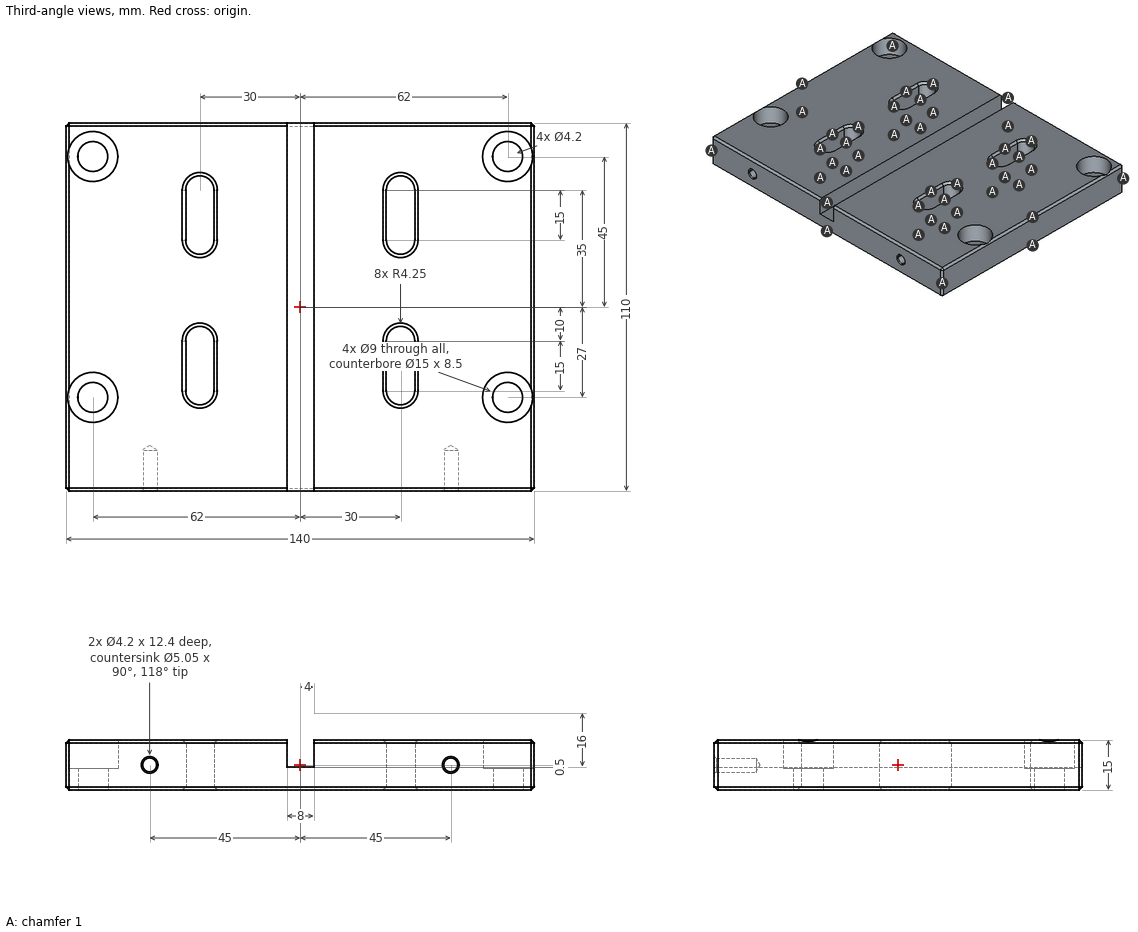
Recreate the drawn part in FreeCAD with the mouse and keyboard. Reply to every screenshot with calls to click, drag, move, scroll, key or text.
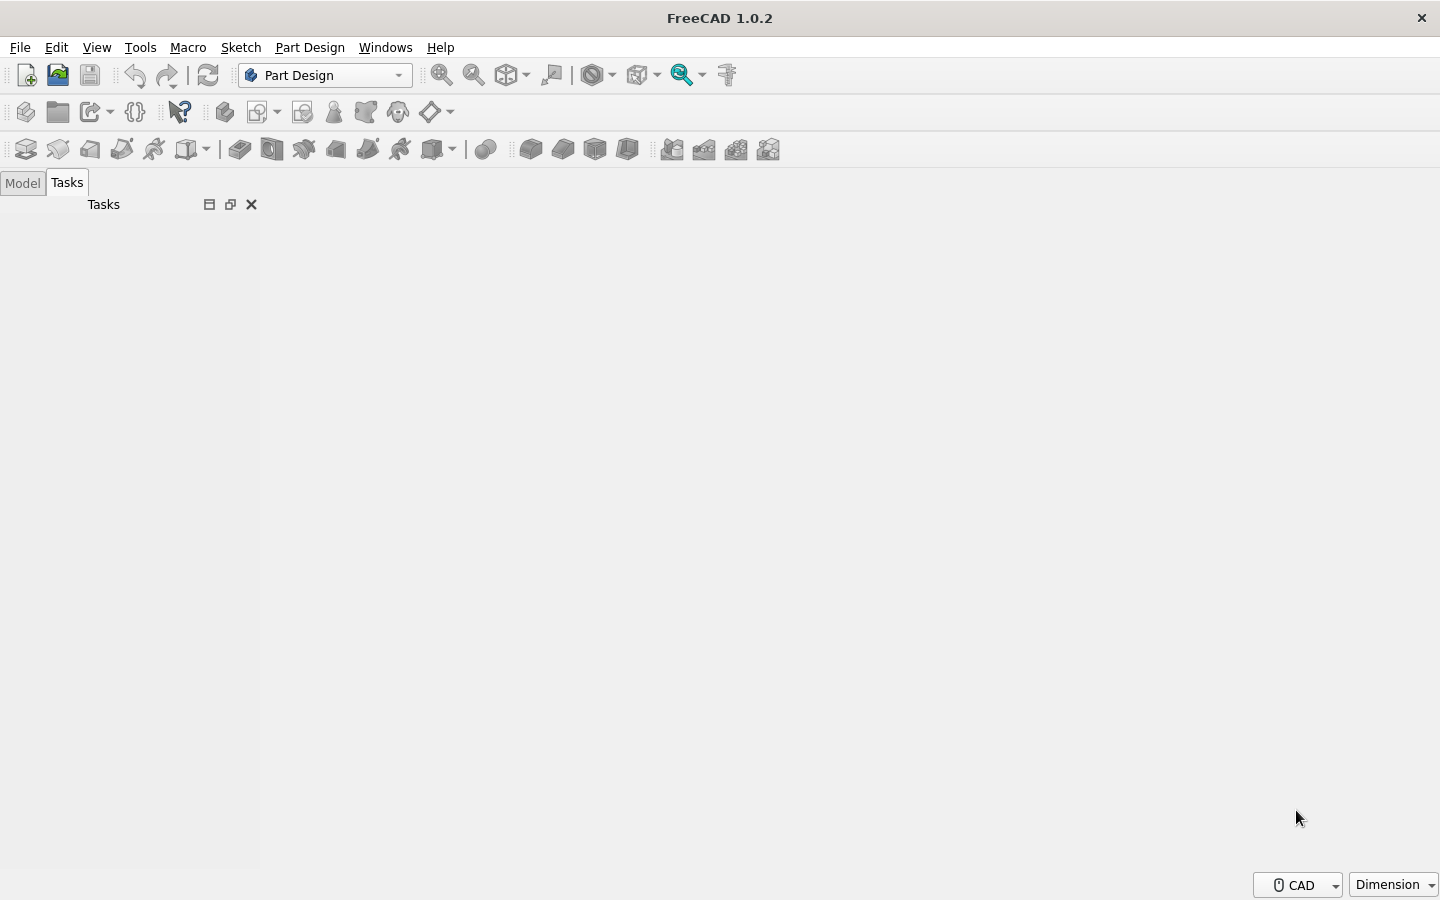
key(ctrl+n)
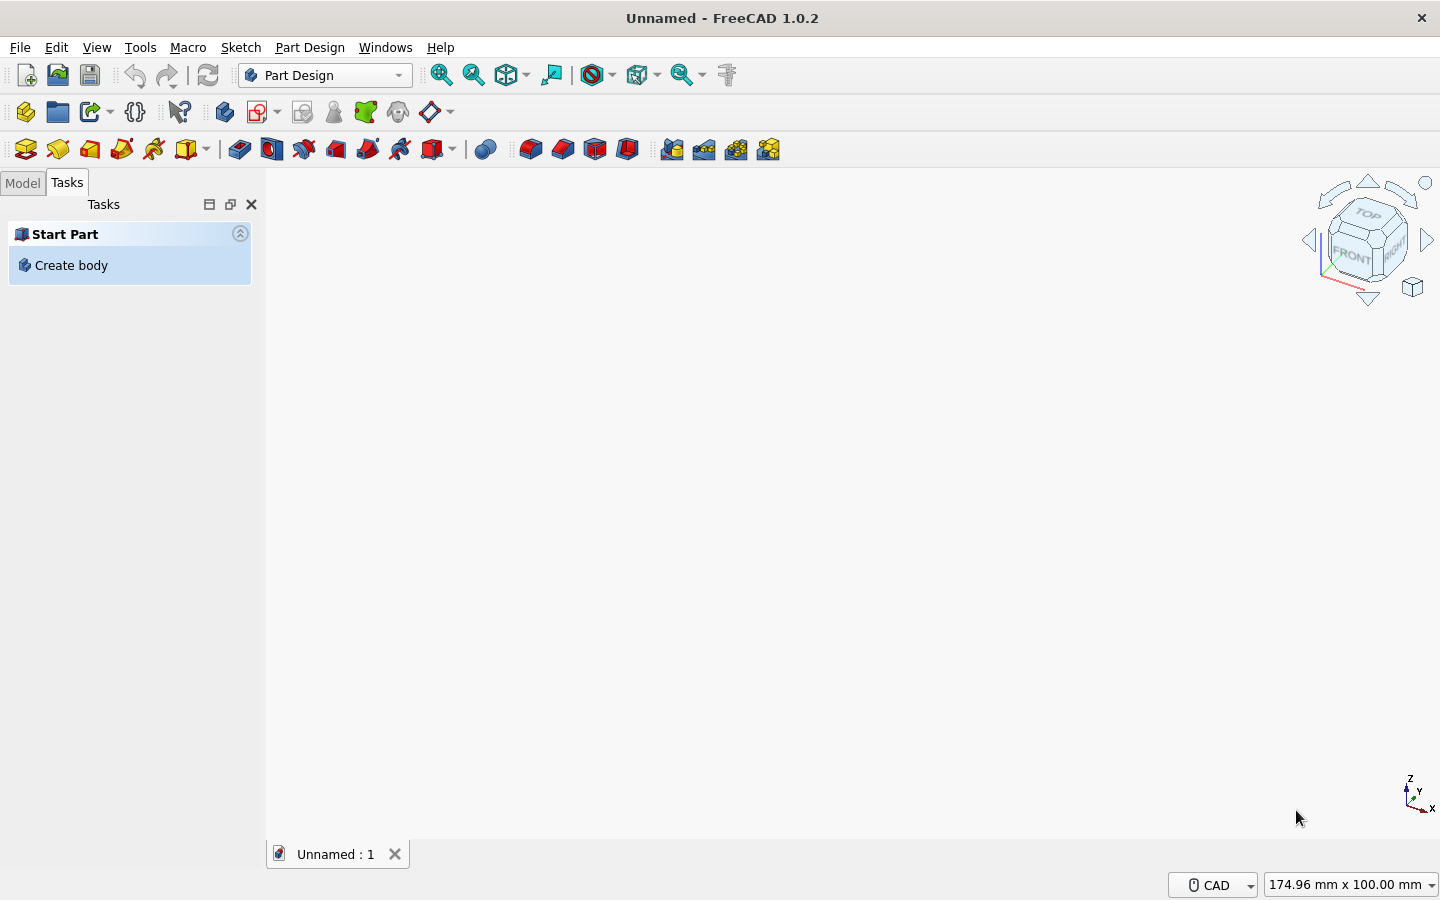
click(258, 112)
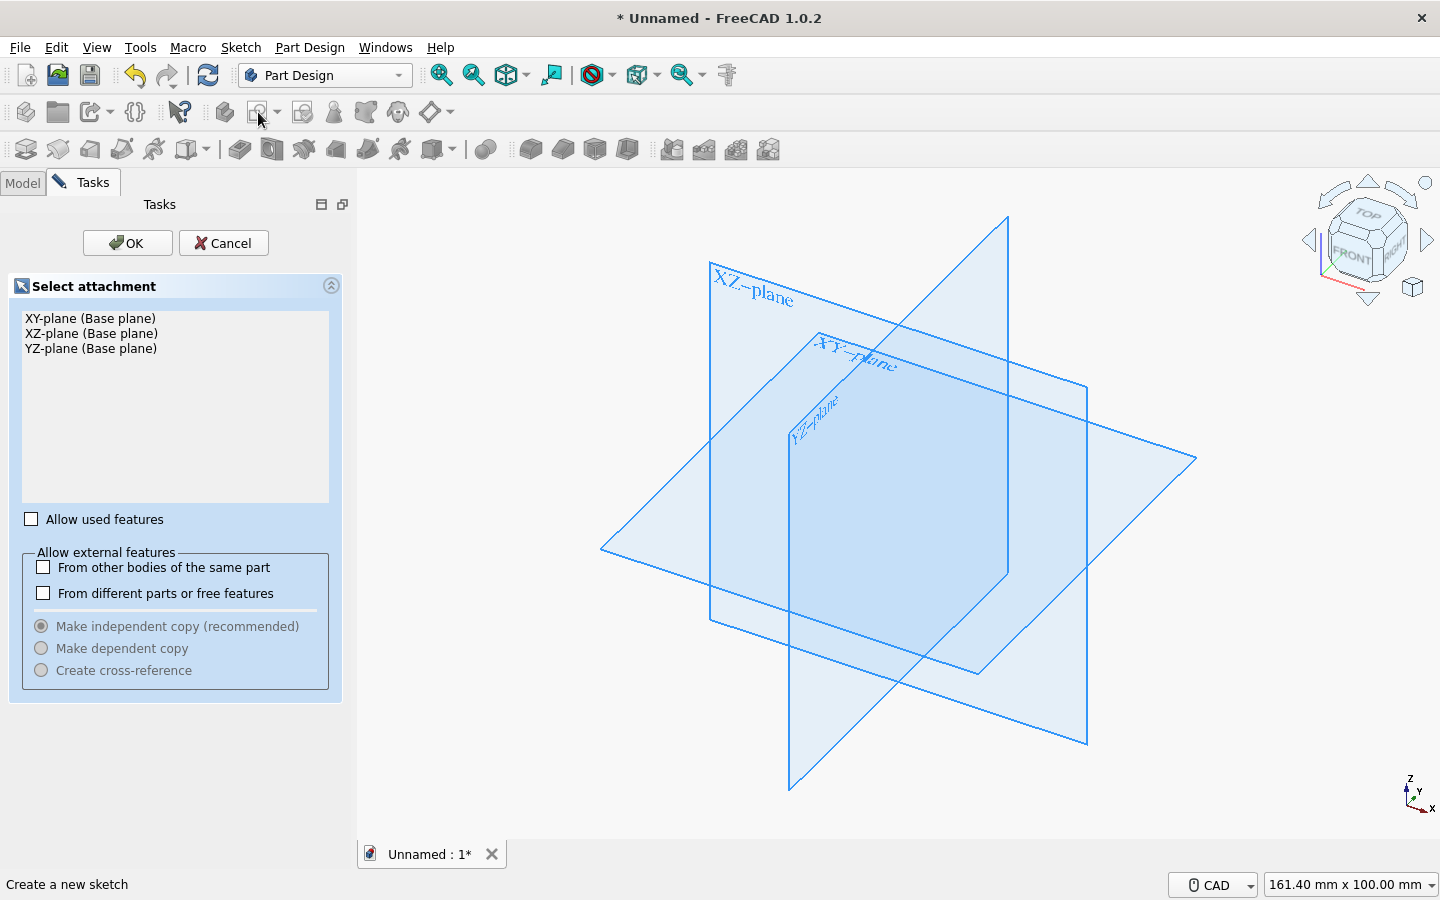
click(82, 318)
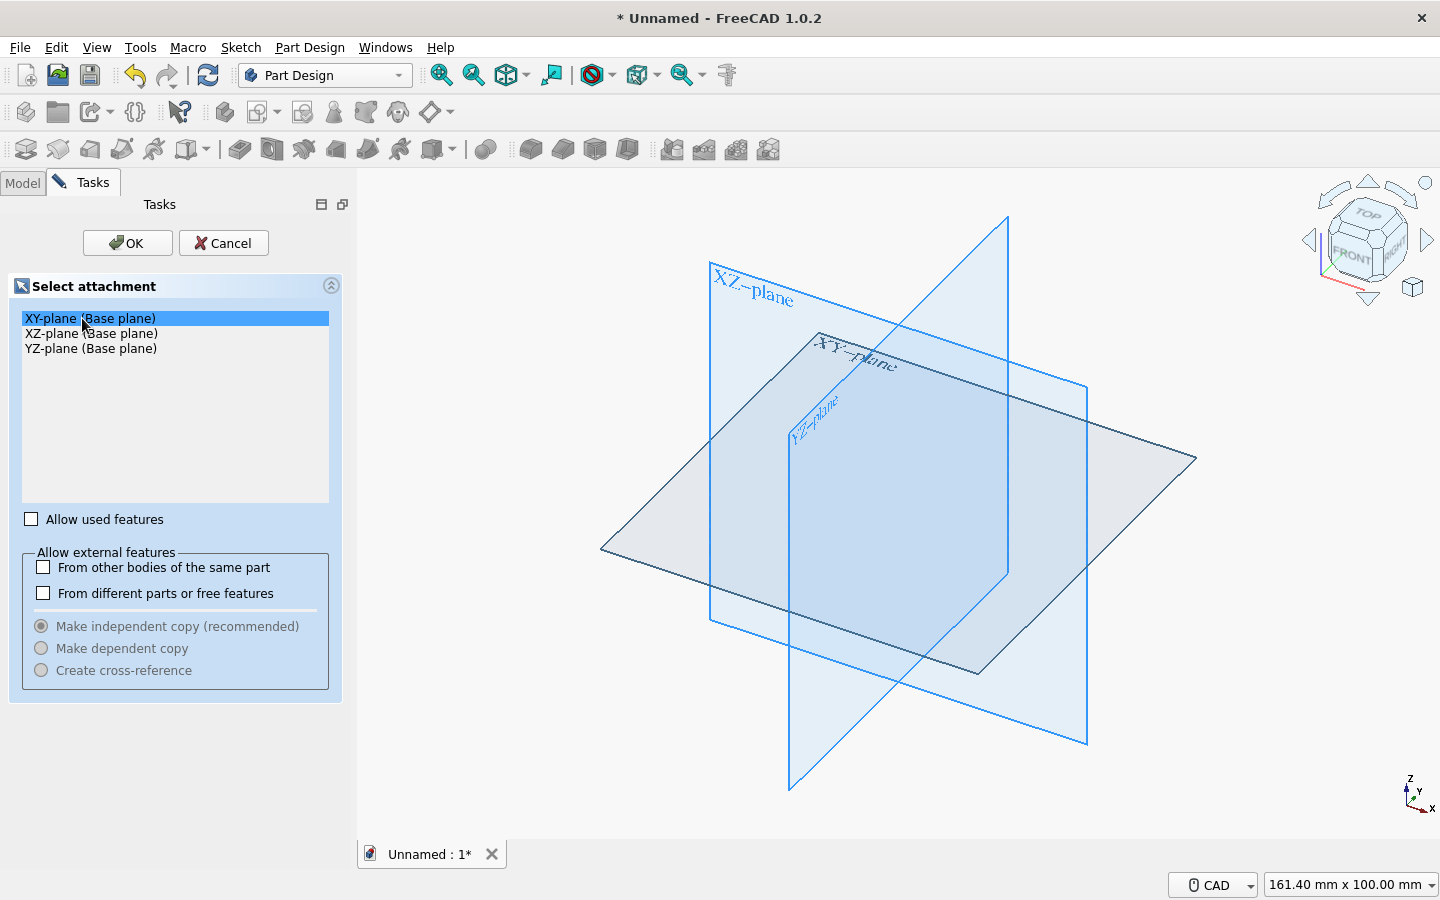
click(128, 243)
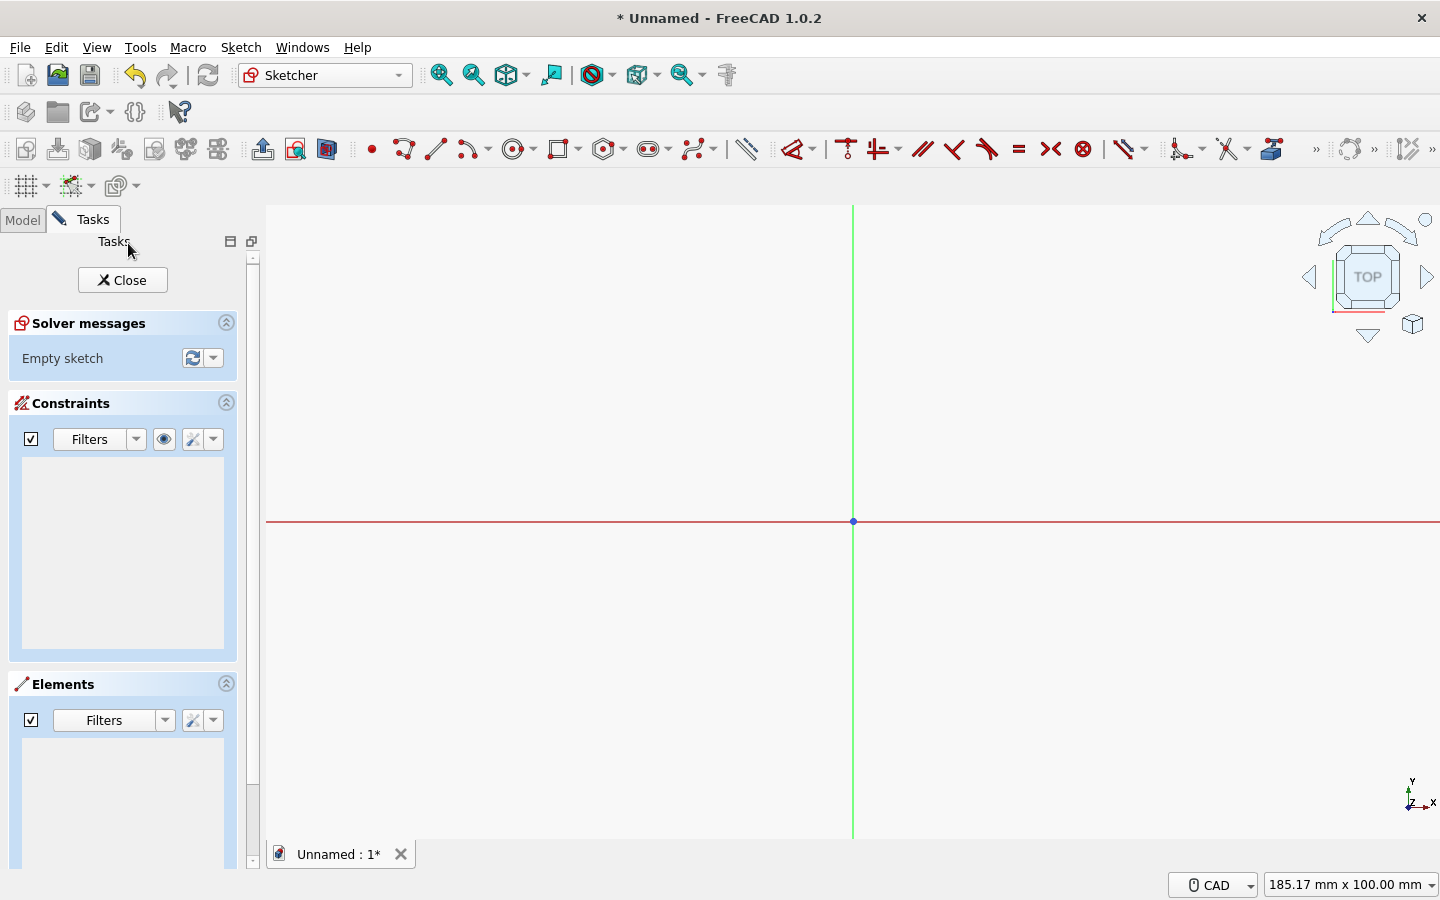
scroll(701, 522, down, 3)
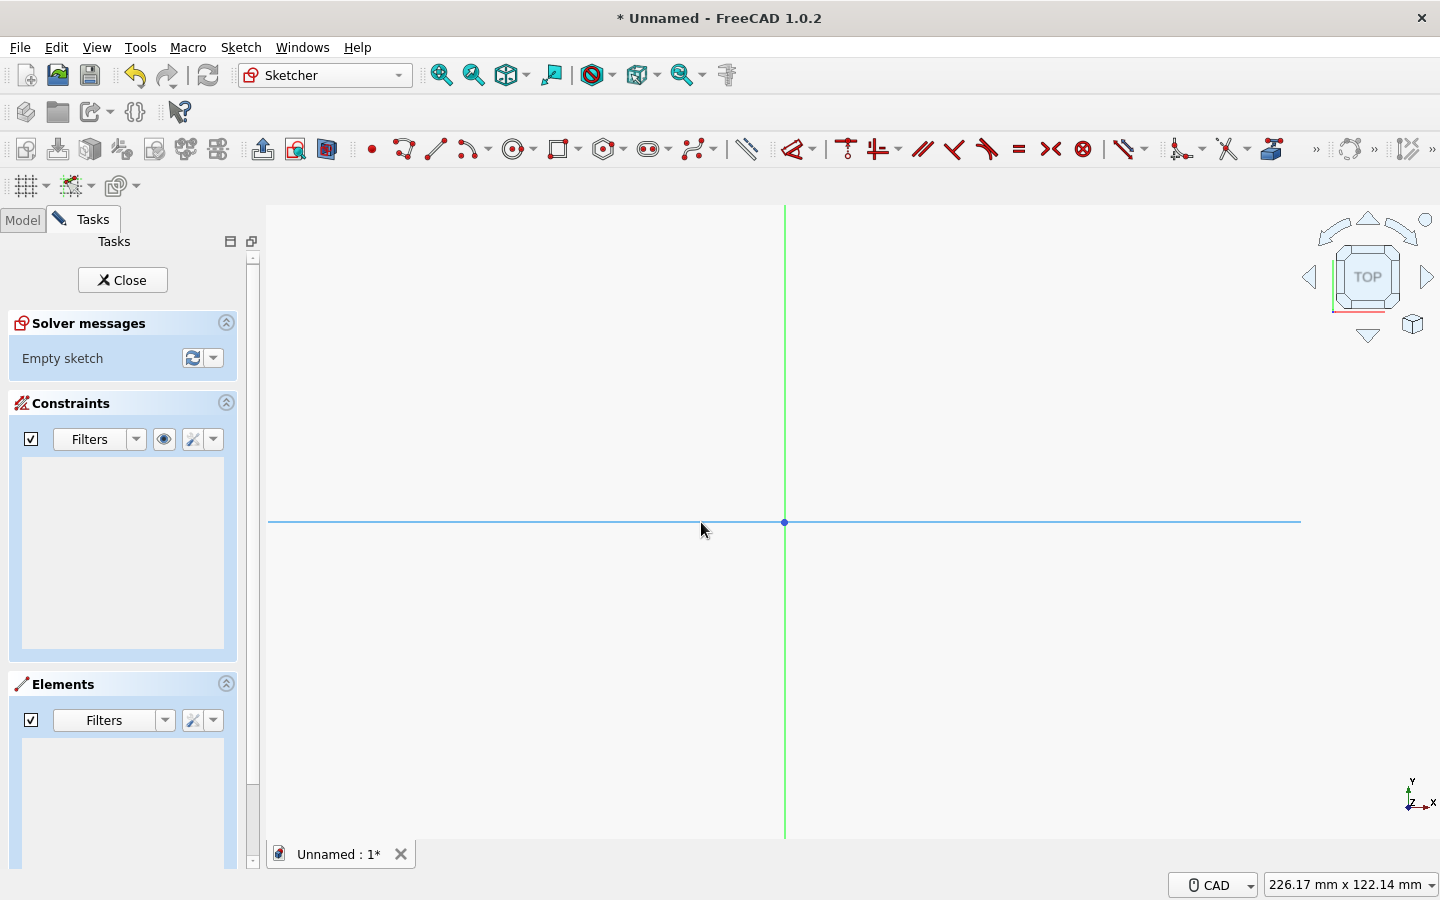
key(g)
key(v)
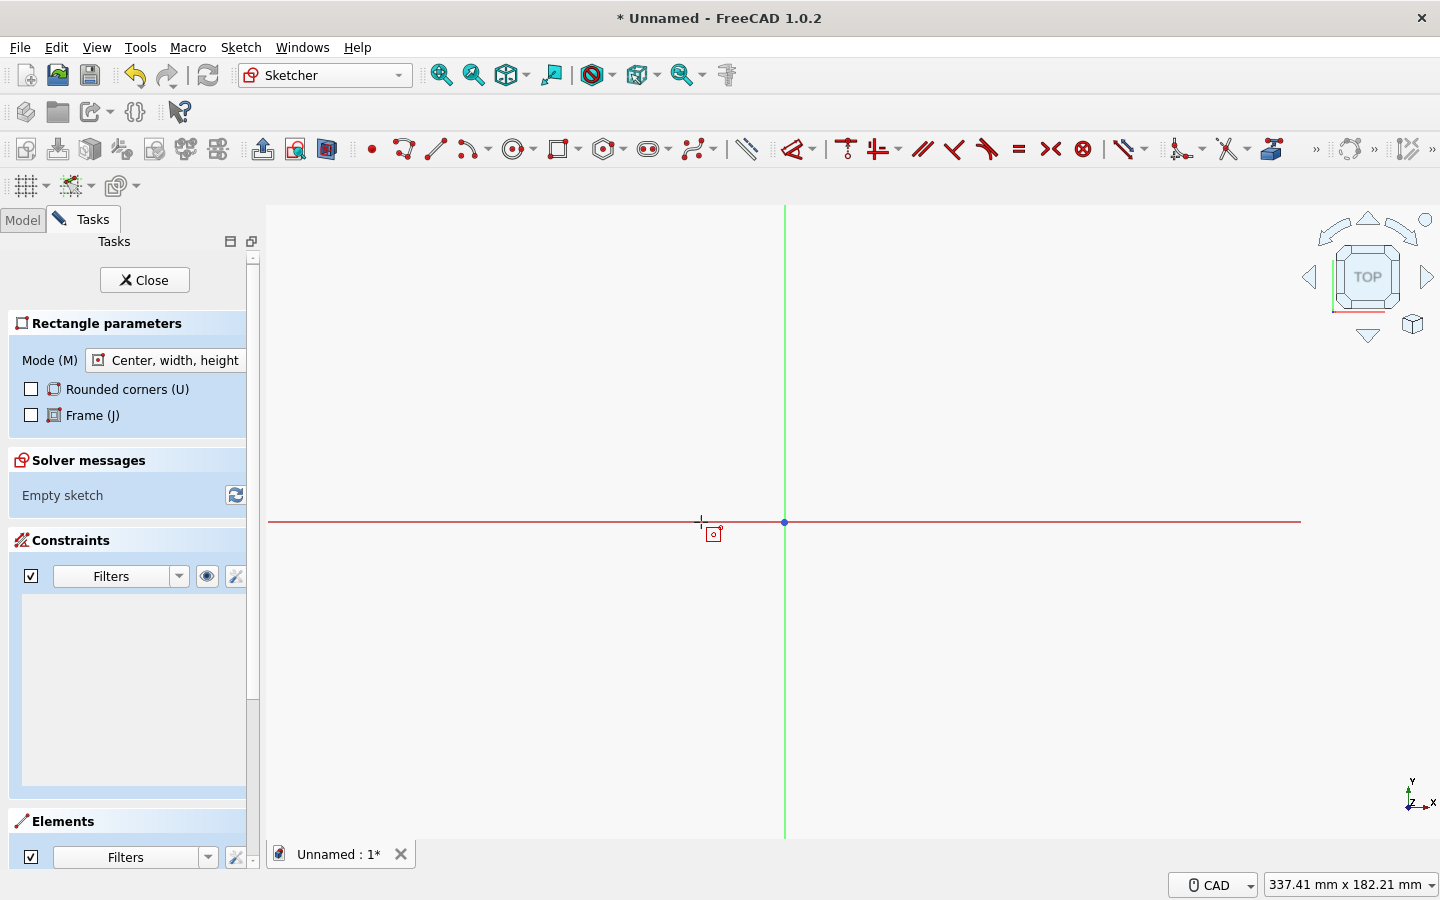
click(785, 522)
click(1028, 331)
key(Escape)